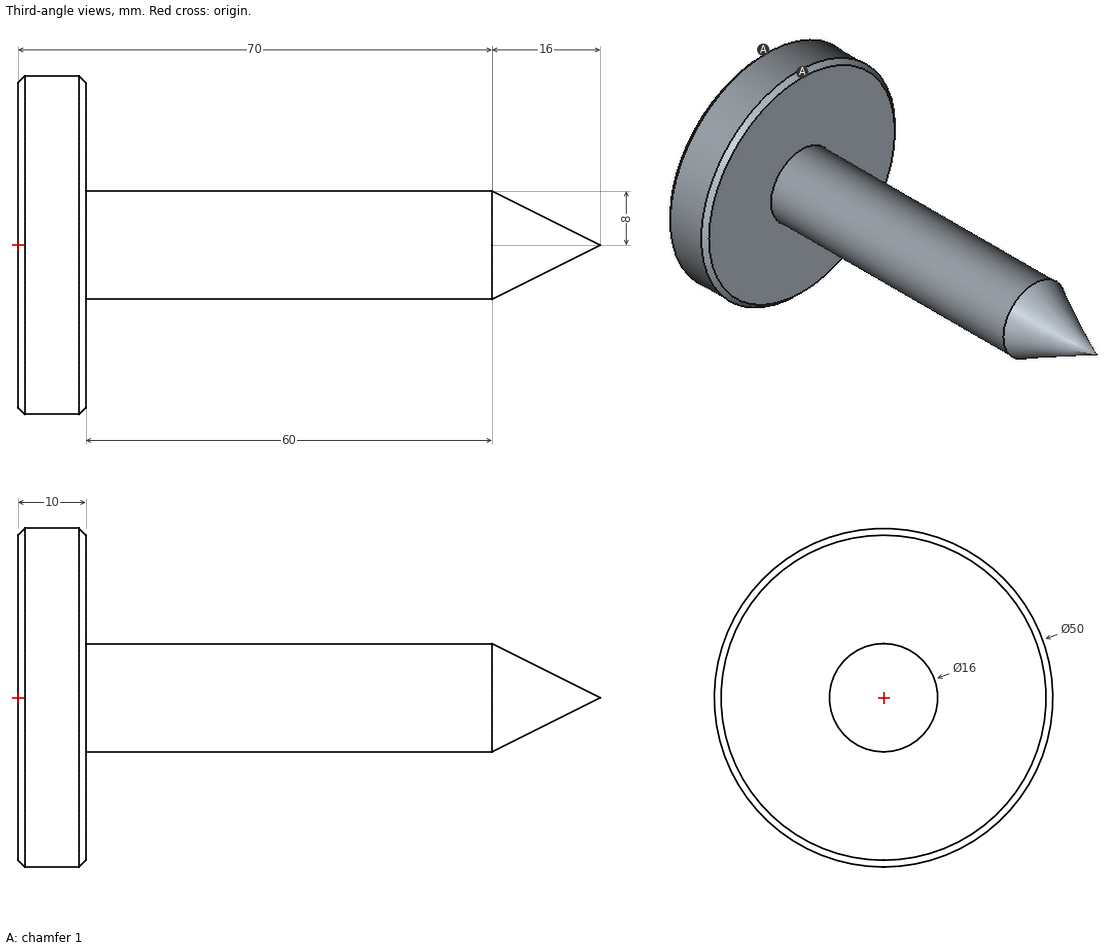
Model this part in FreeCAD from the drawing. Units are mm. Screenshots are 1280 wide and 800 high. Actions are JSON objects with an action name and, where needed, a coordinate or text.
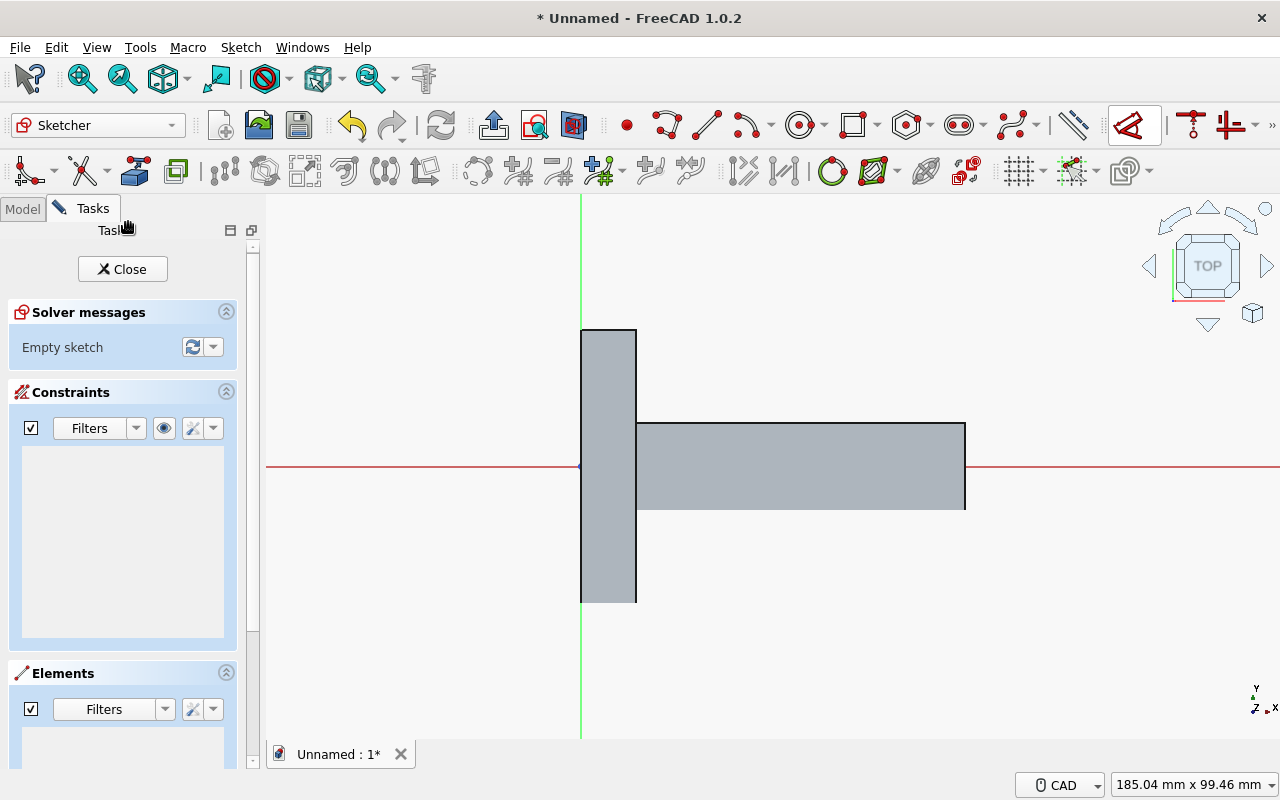
{"action": "key", "text": "q s"}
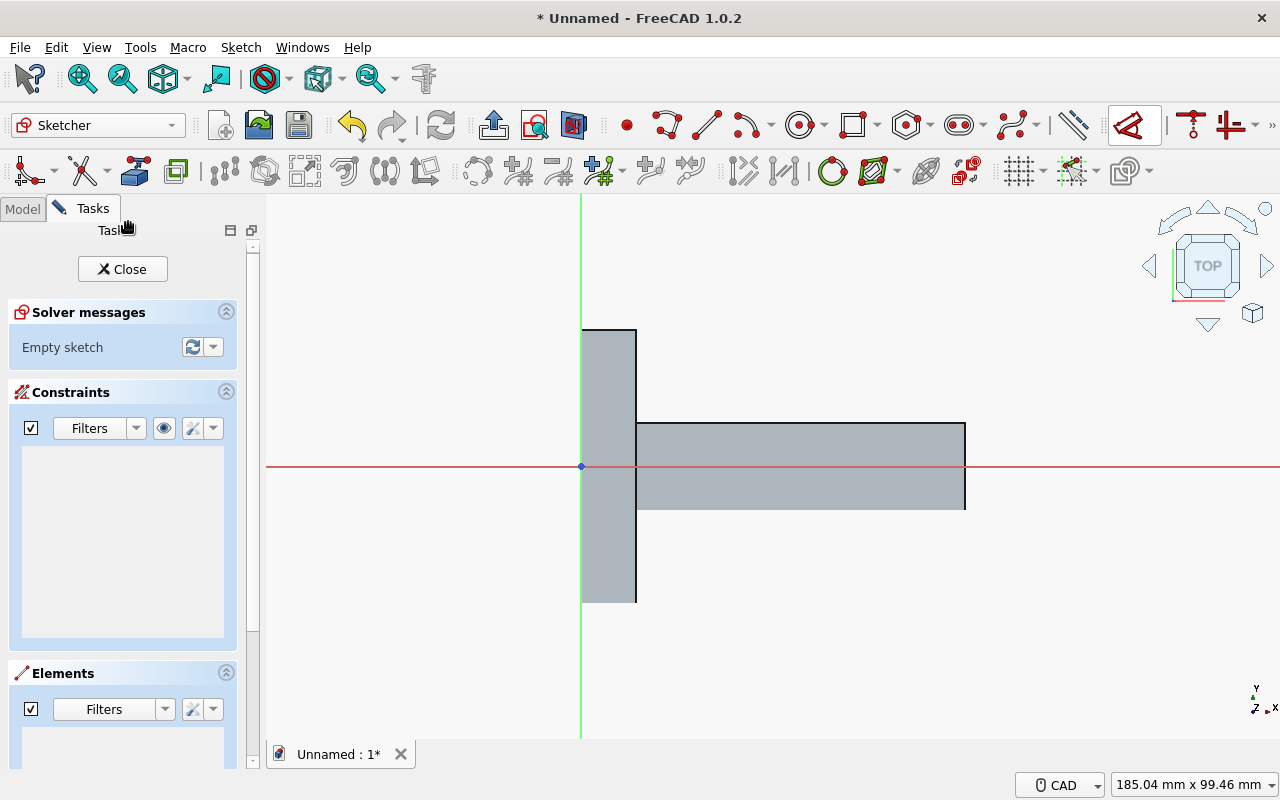
{"action": "scroll", "coordinate": [1069, 440], "scroll_direction": "up", "scroll_amount": 9}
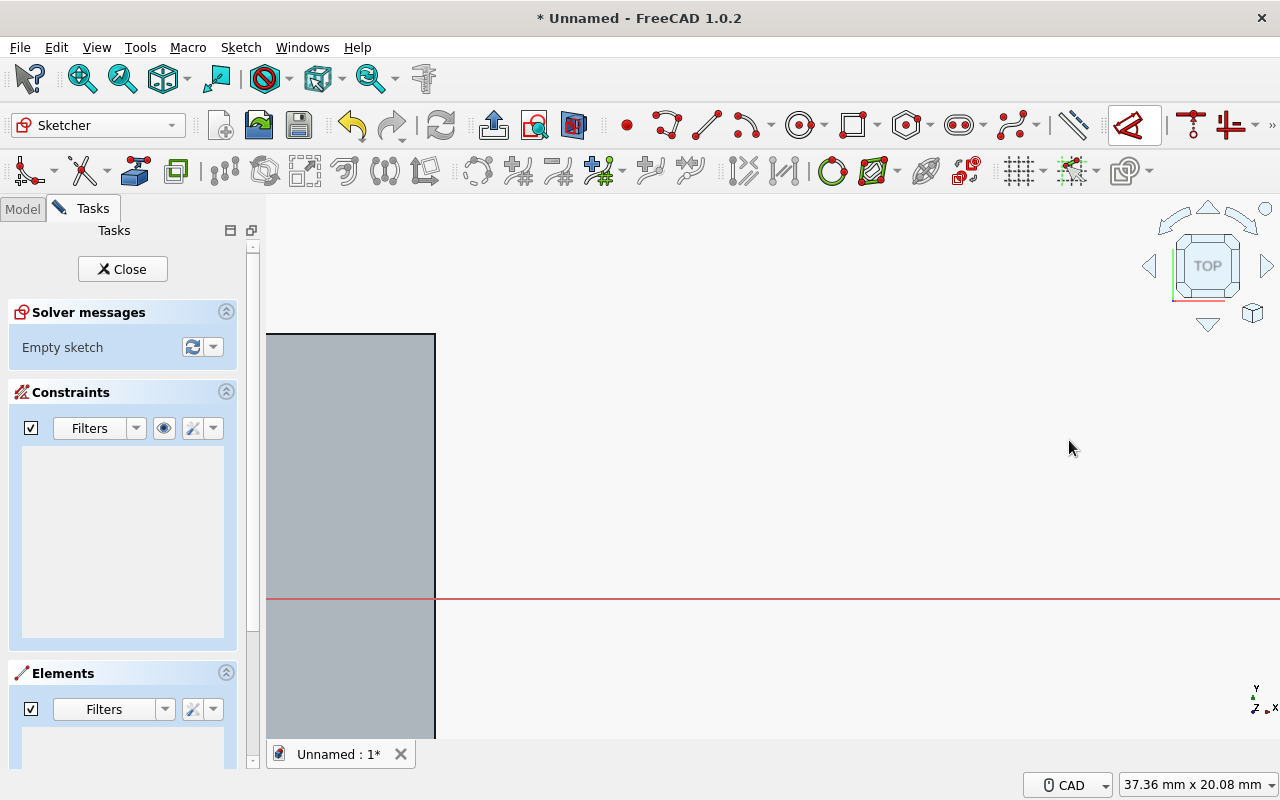
{"action": "left_click", "coordinate": [668, 126]}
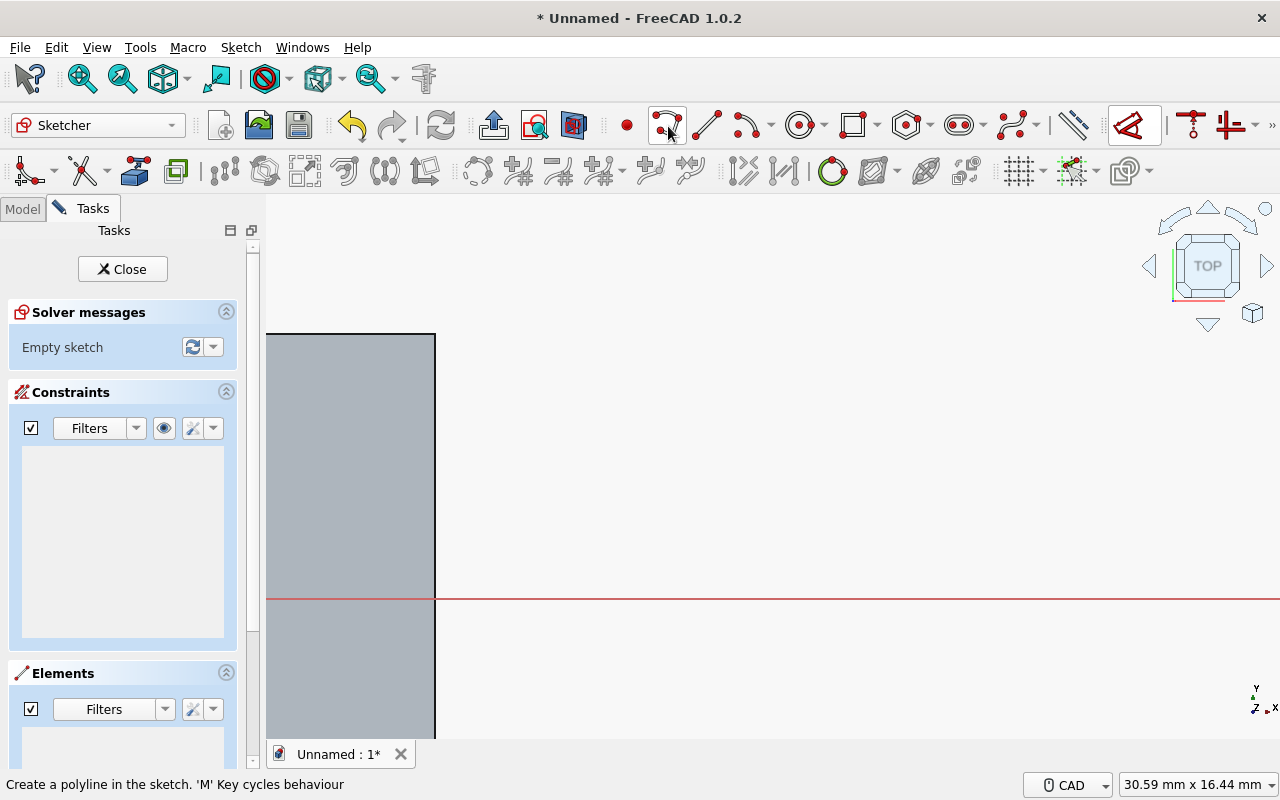
{"action": "left_click", "coordinate": [435, 599]}
{"action": "left_click", "coordinate": [965, 590]}
{"action": "left_click", "coordinate": [435, 334]}
{"action": "left_click", "coordinate": [435, 599]}
{"action": "key", "text": "Escape"}
{"action": "key", "text": "Escape"}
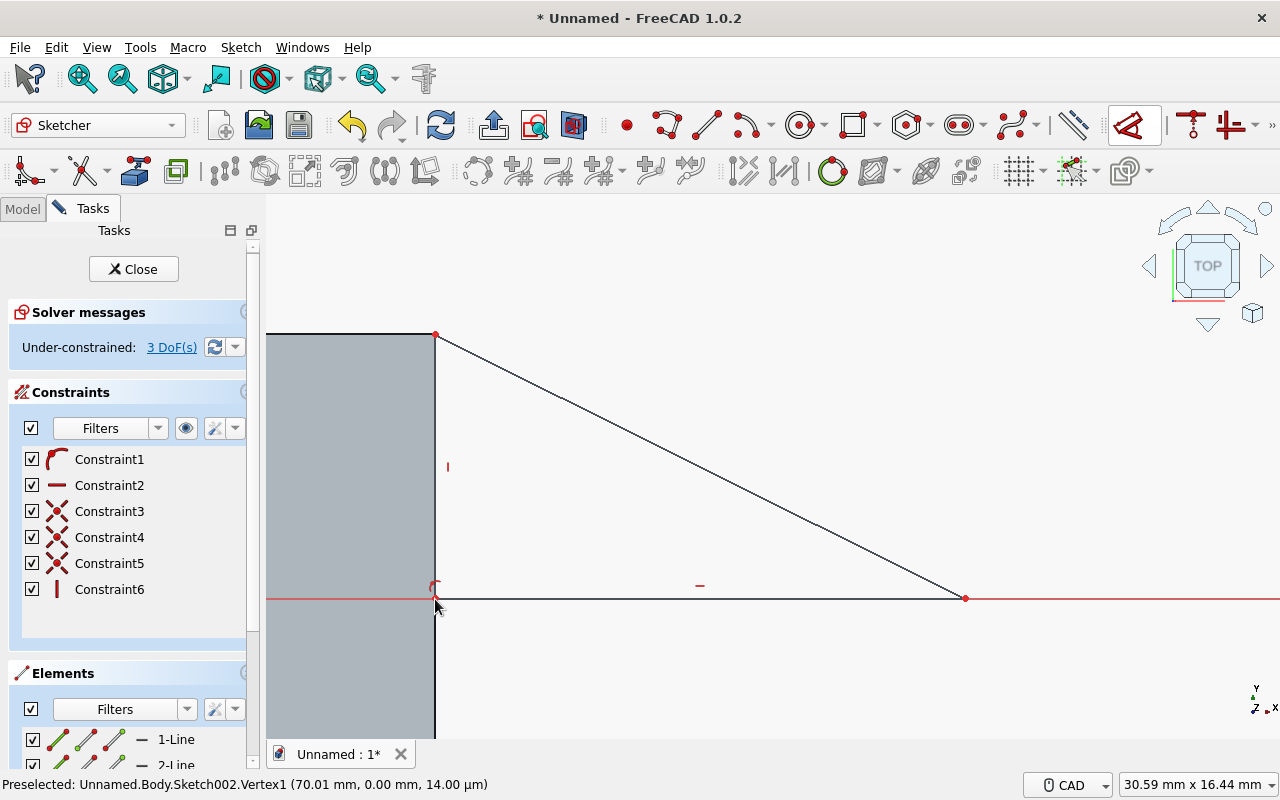
{"action": "left_click", "coordinate": [435, 414]}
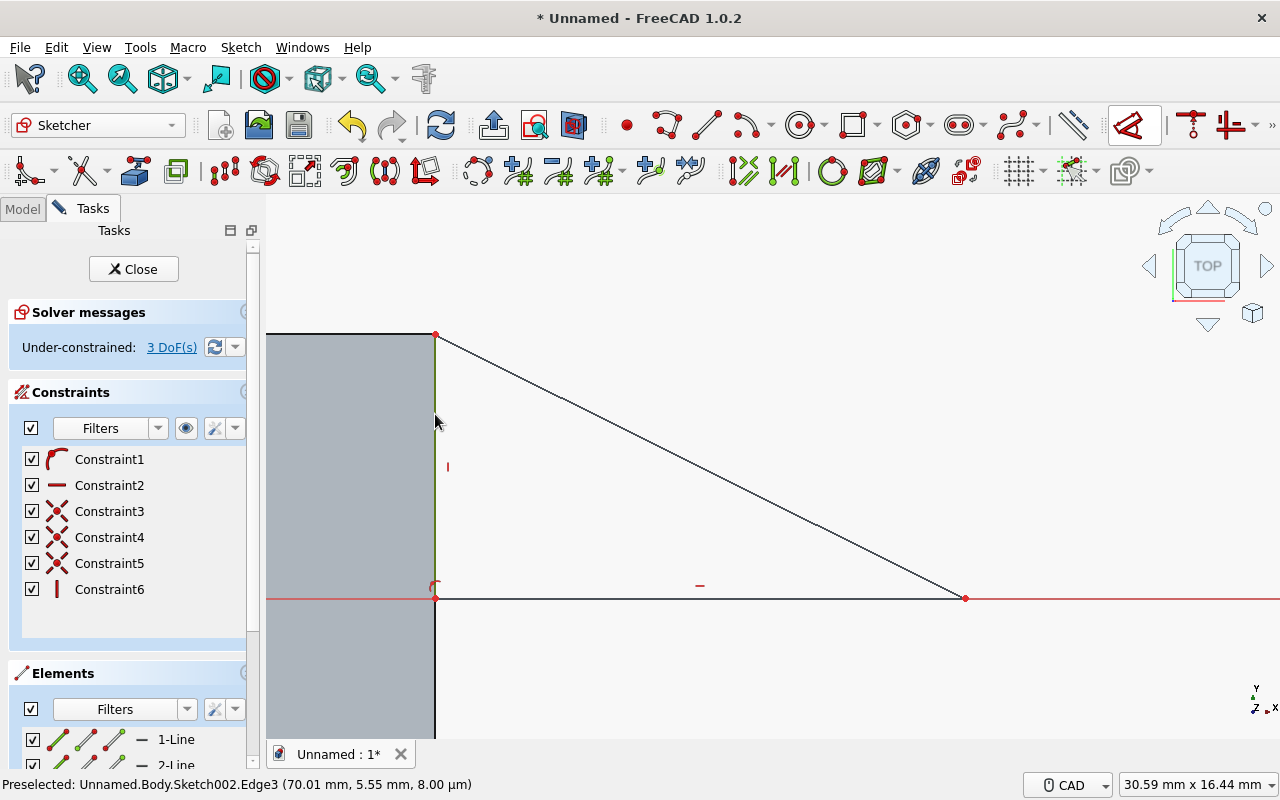
{"action": "key", "text": "i"}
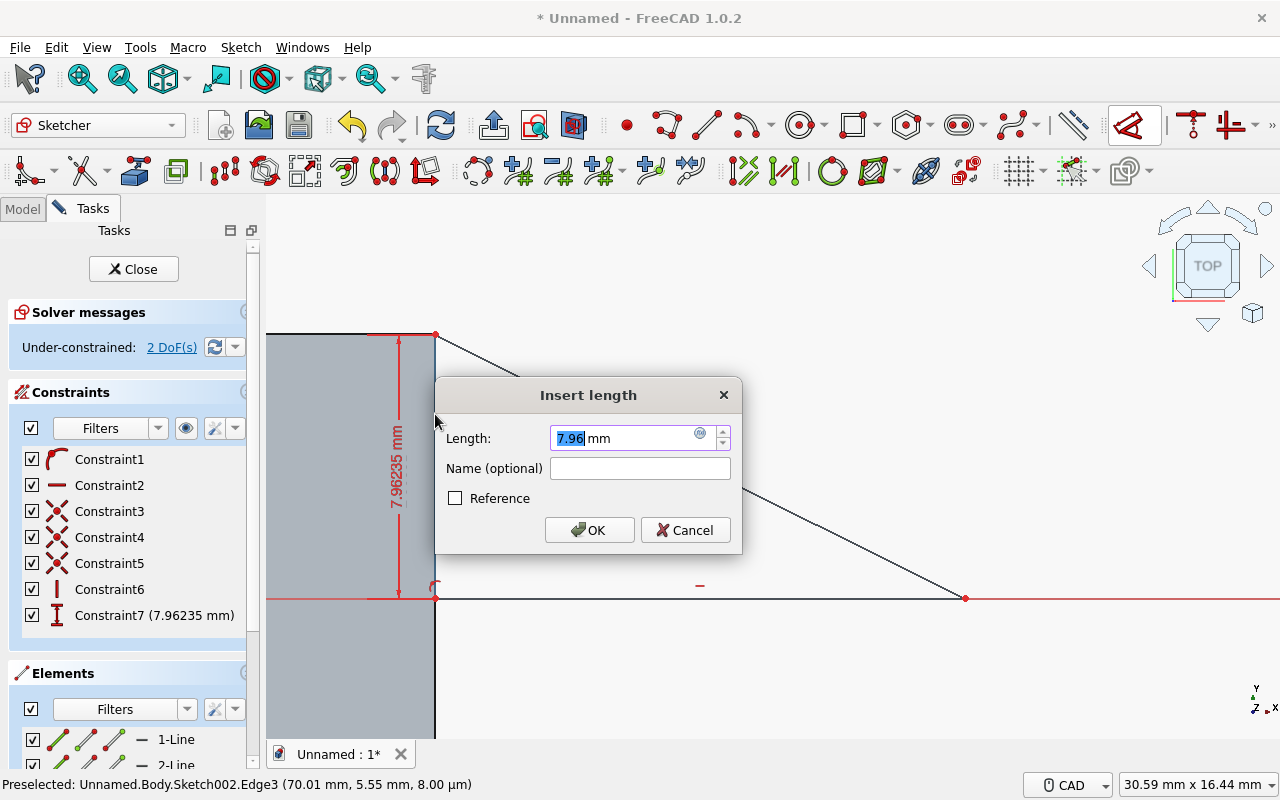
{"action": "type", "text": "8"}
{"action": "key", "text": "Return"}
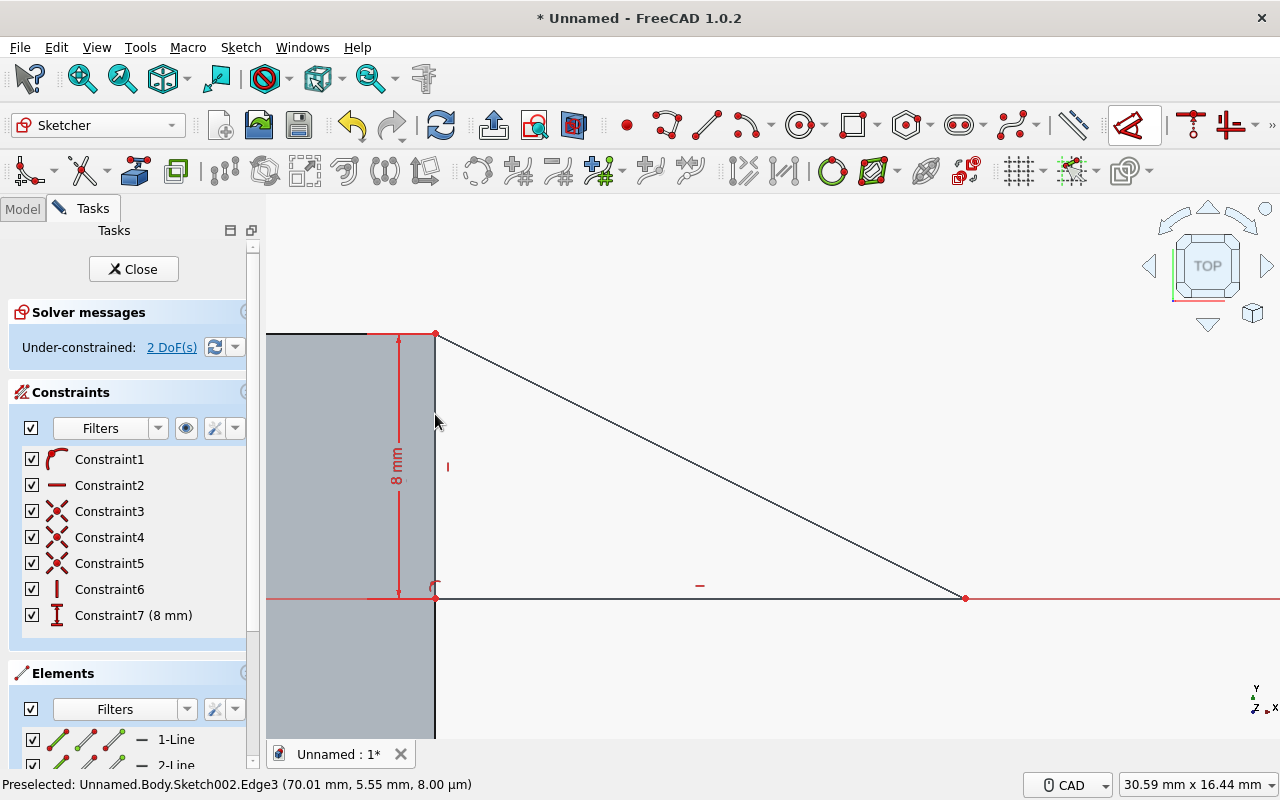
{"action": "left_click", "coordinate": [594, 599]}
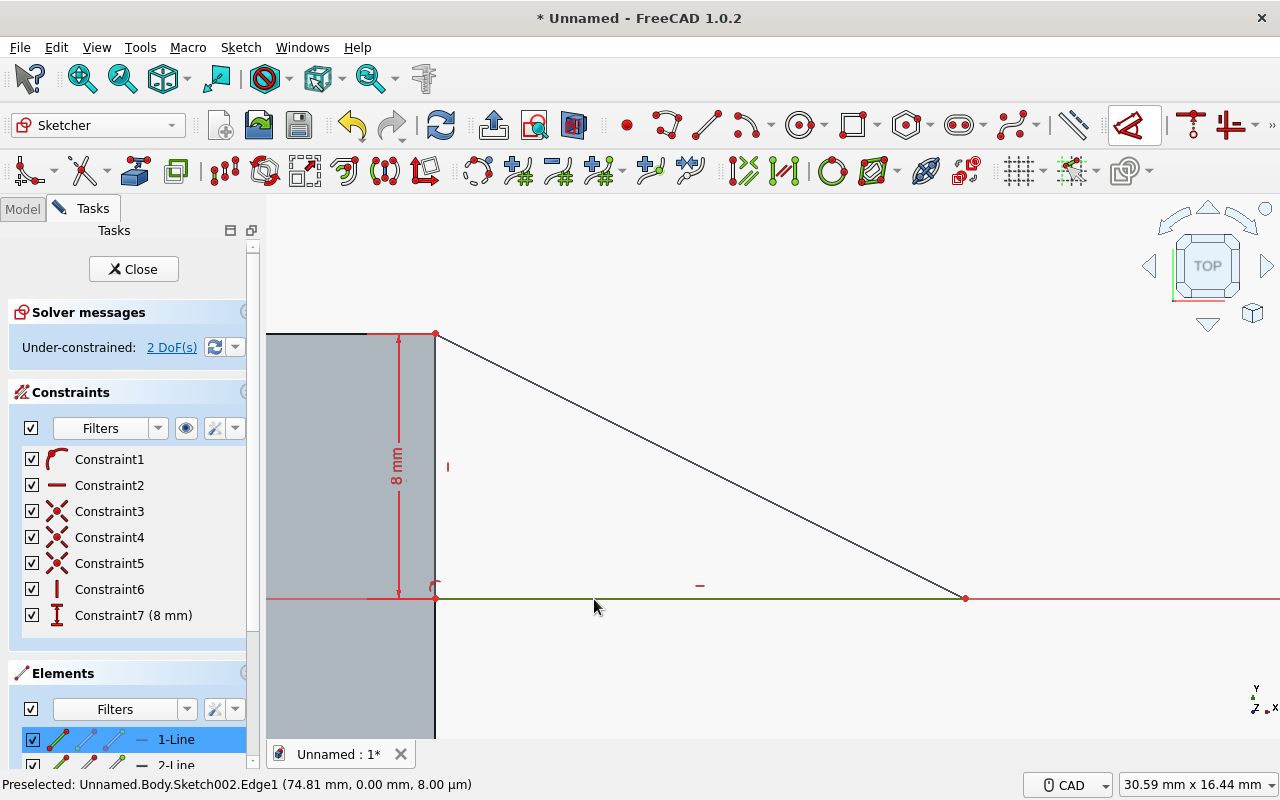
{"action": "key", "text": "l"}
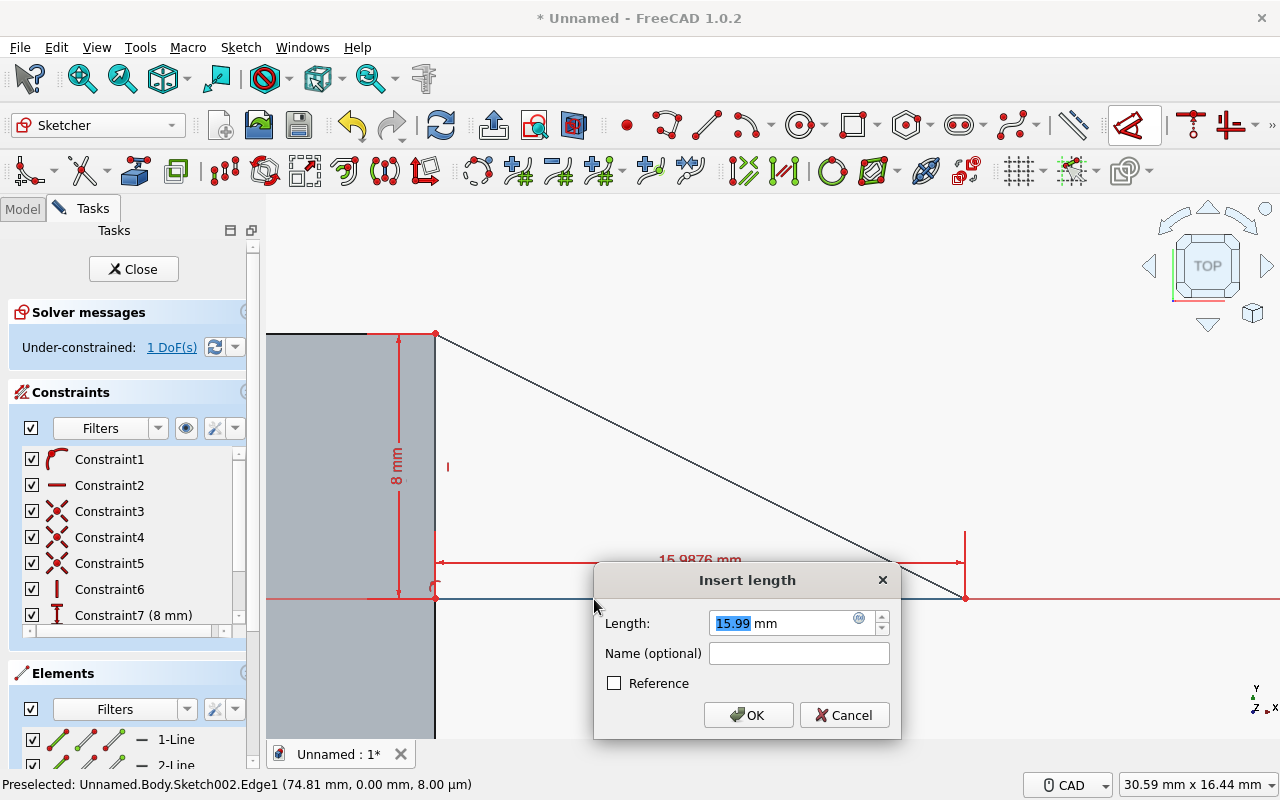
{"action": "type", "text": "16"}
{"action": "key", "text": "Return"}